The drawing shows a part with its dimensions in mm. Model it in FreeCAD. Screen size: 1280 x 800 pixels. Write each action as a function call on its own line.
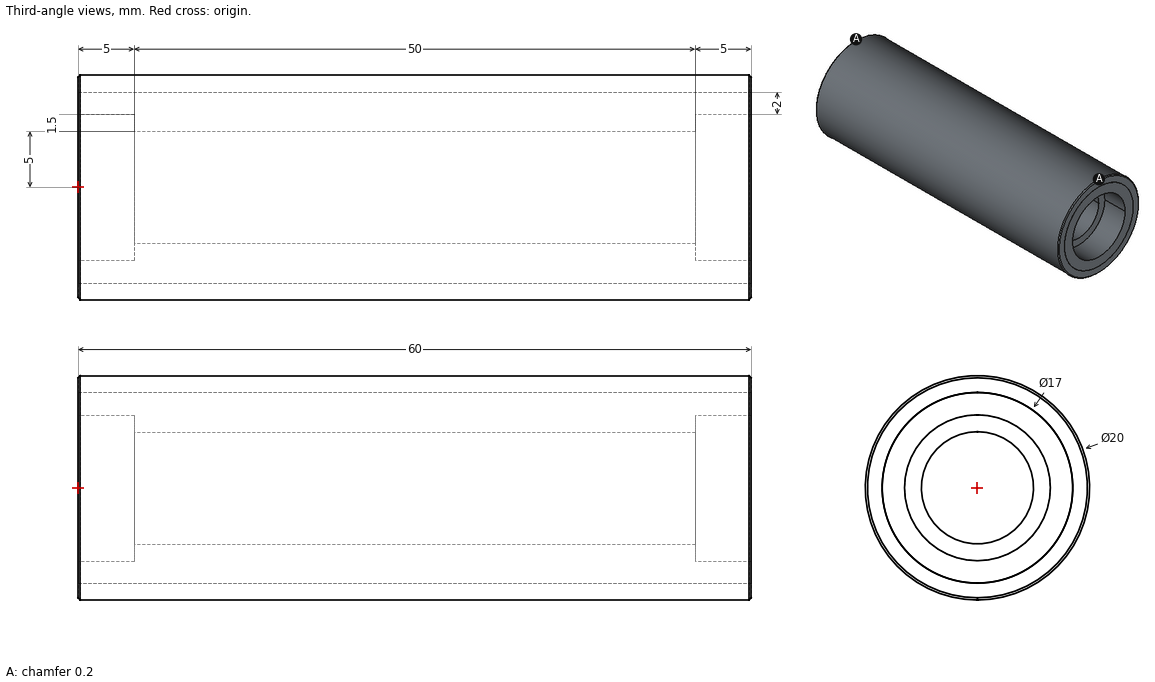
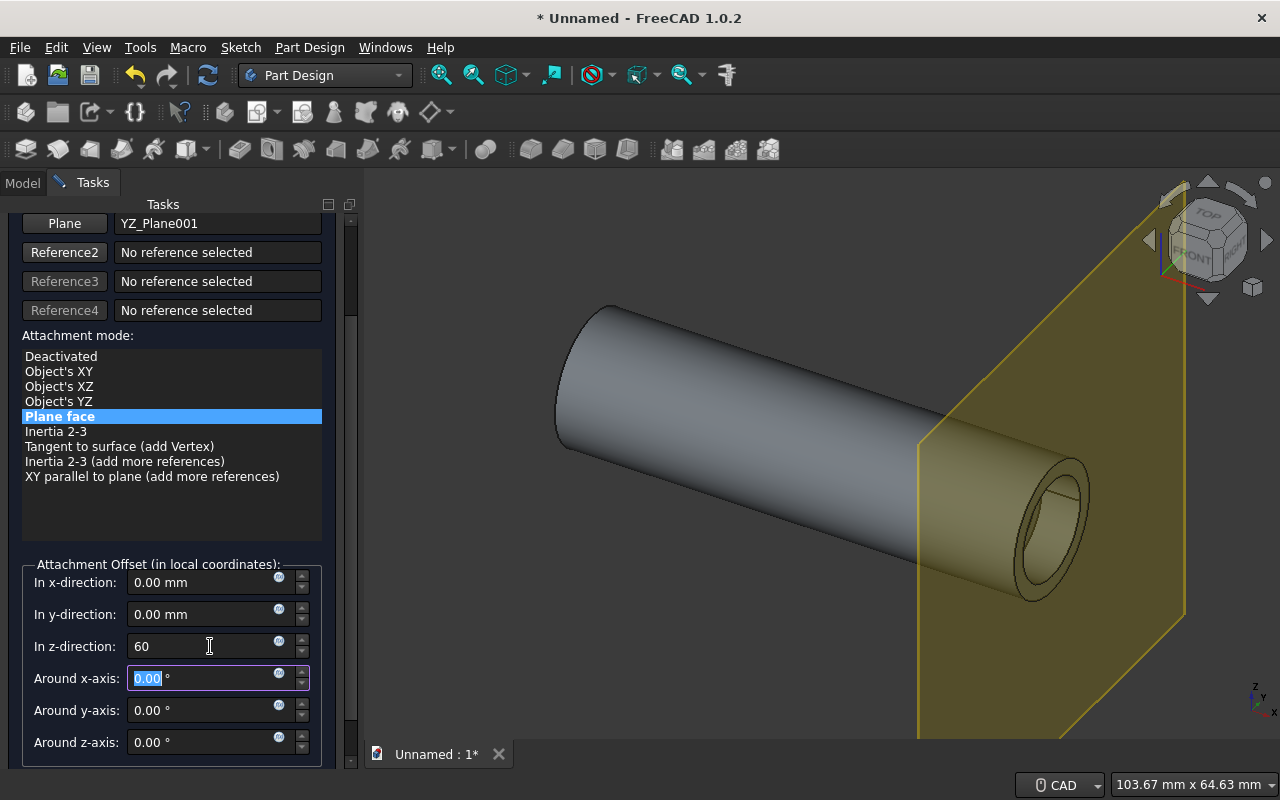
scroll(351, 491, up, 3)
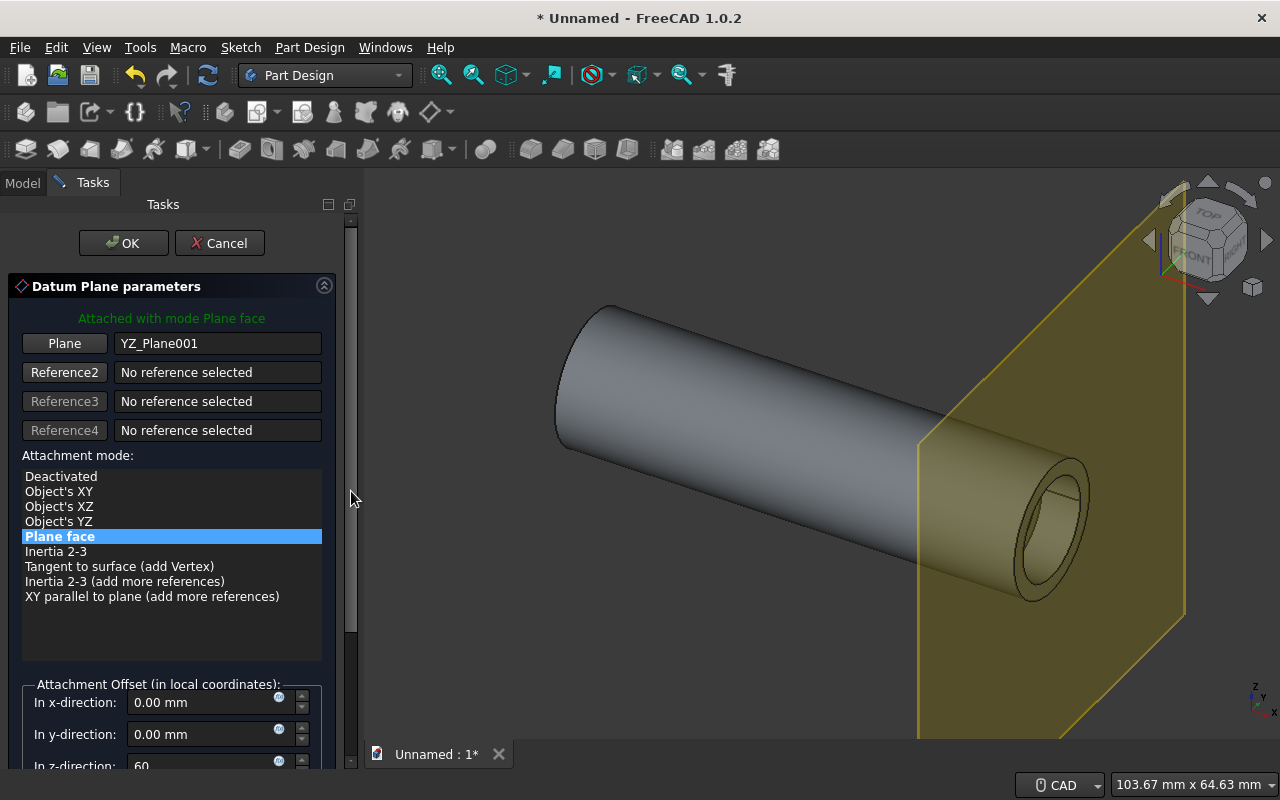
click(124, 243)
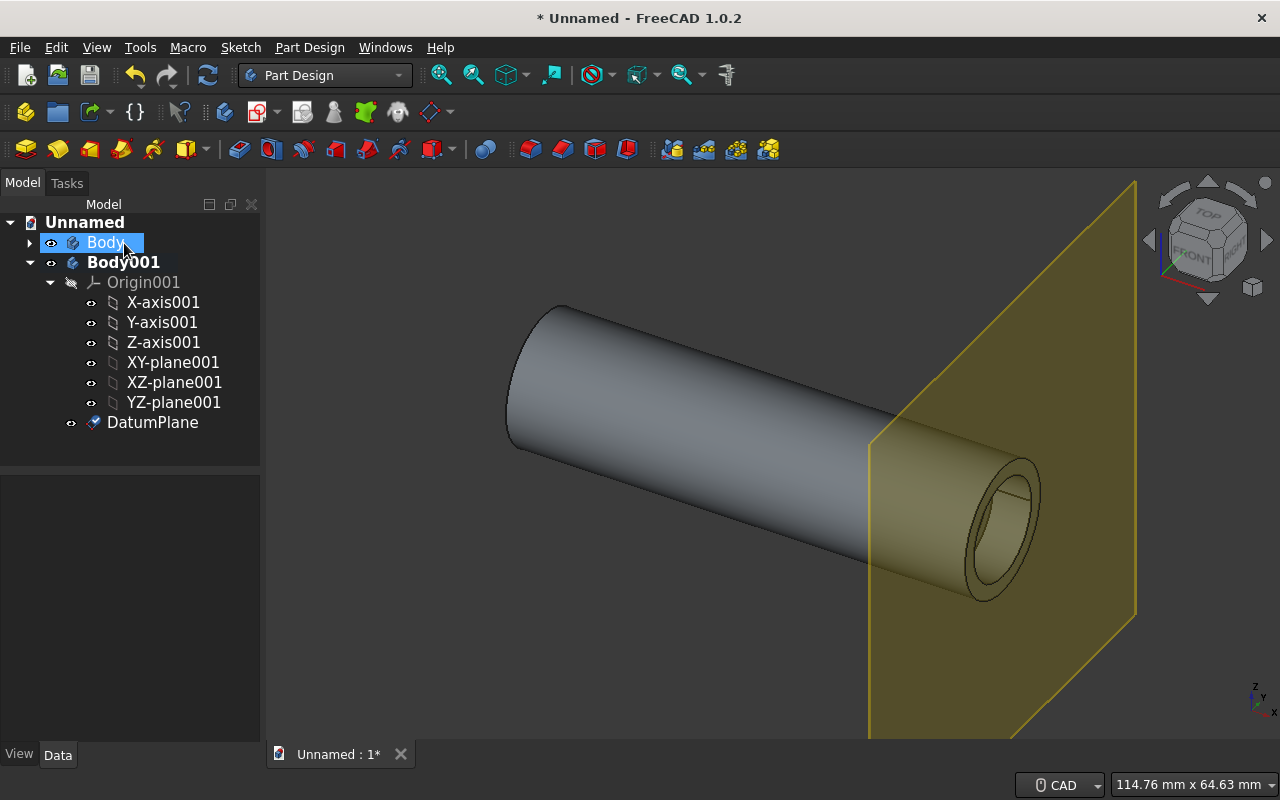
click(116, 423)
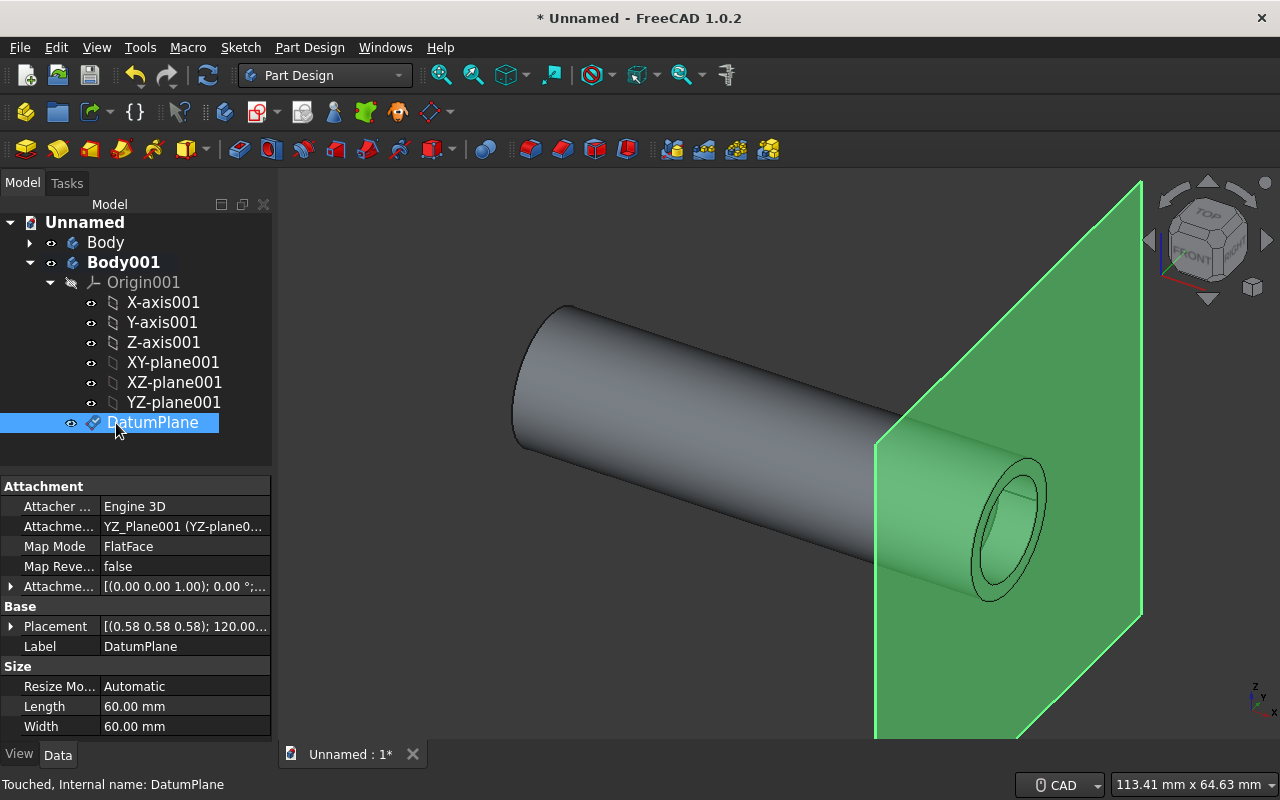
click(258, 112)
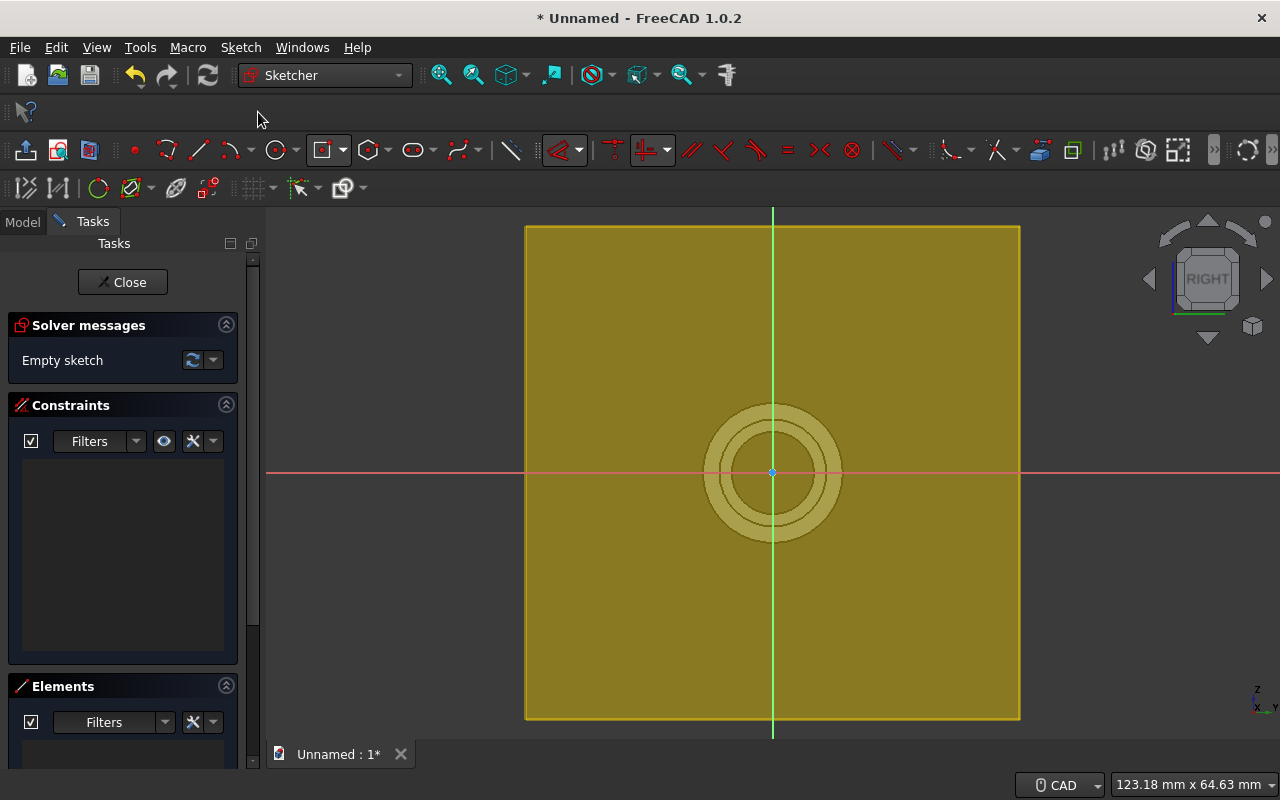
scroll(829, 473, up, 4)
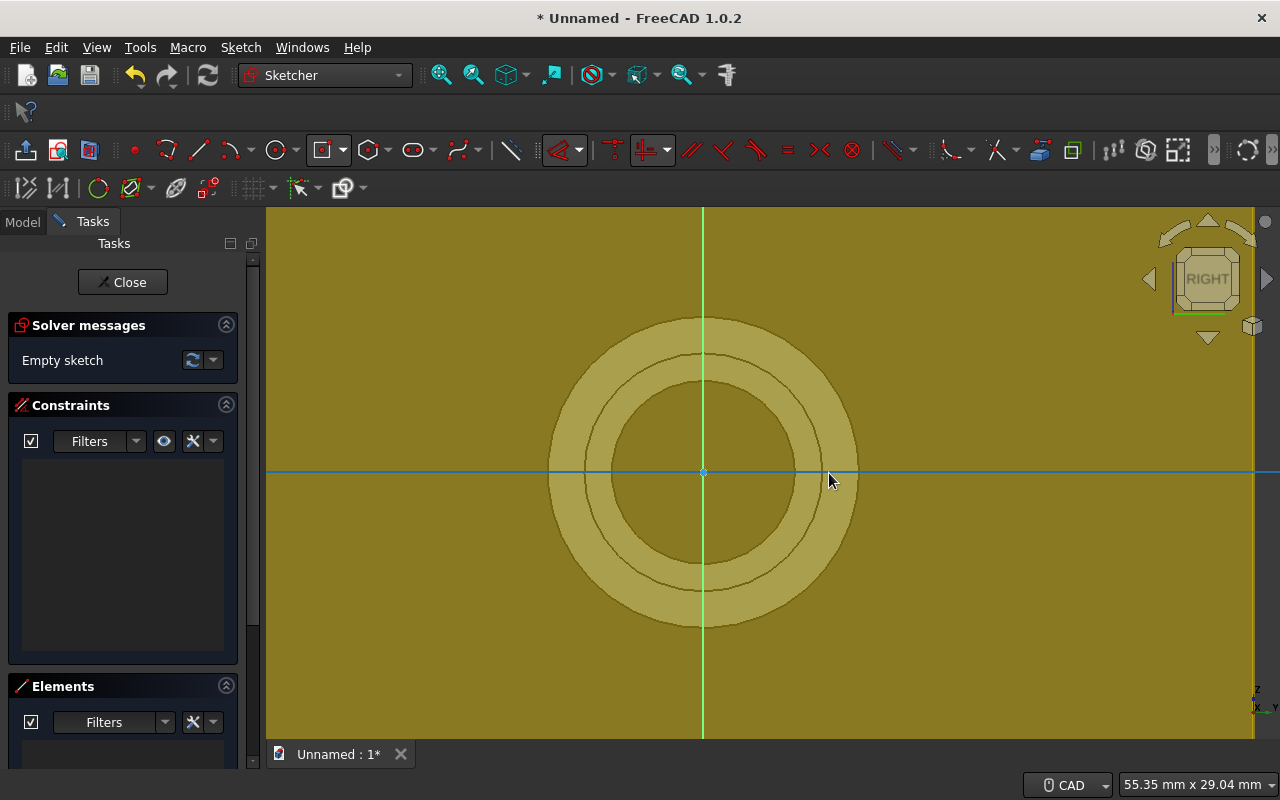
click(276, 150)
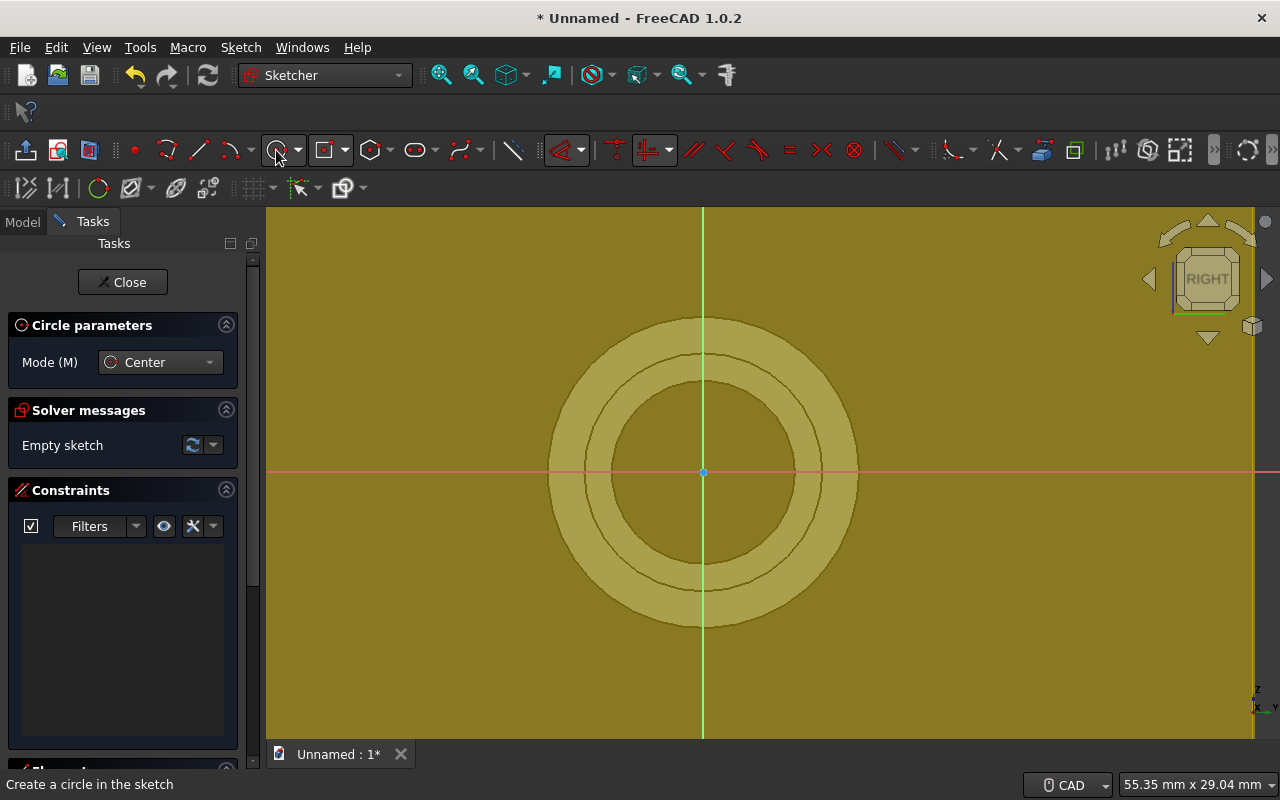
click(703, 472)
move(833, 343)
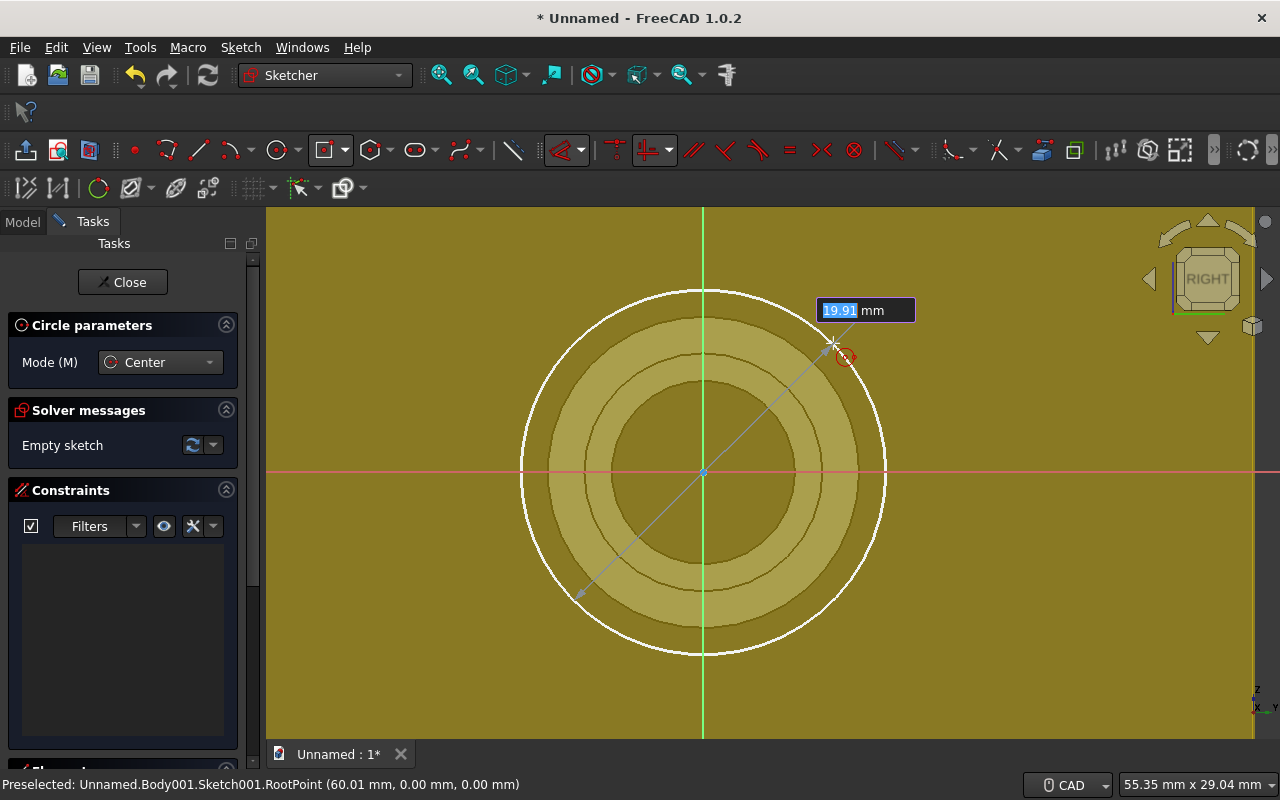
text(20)
key(Return)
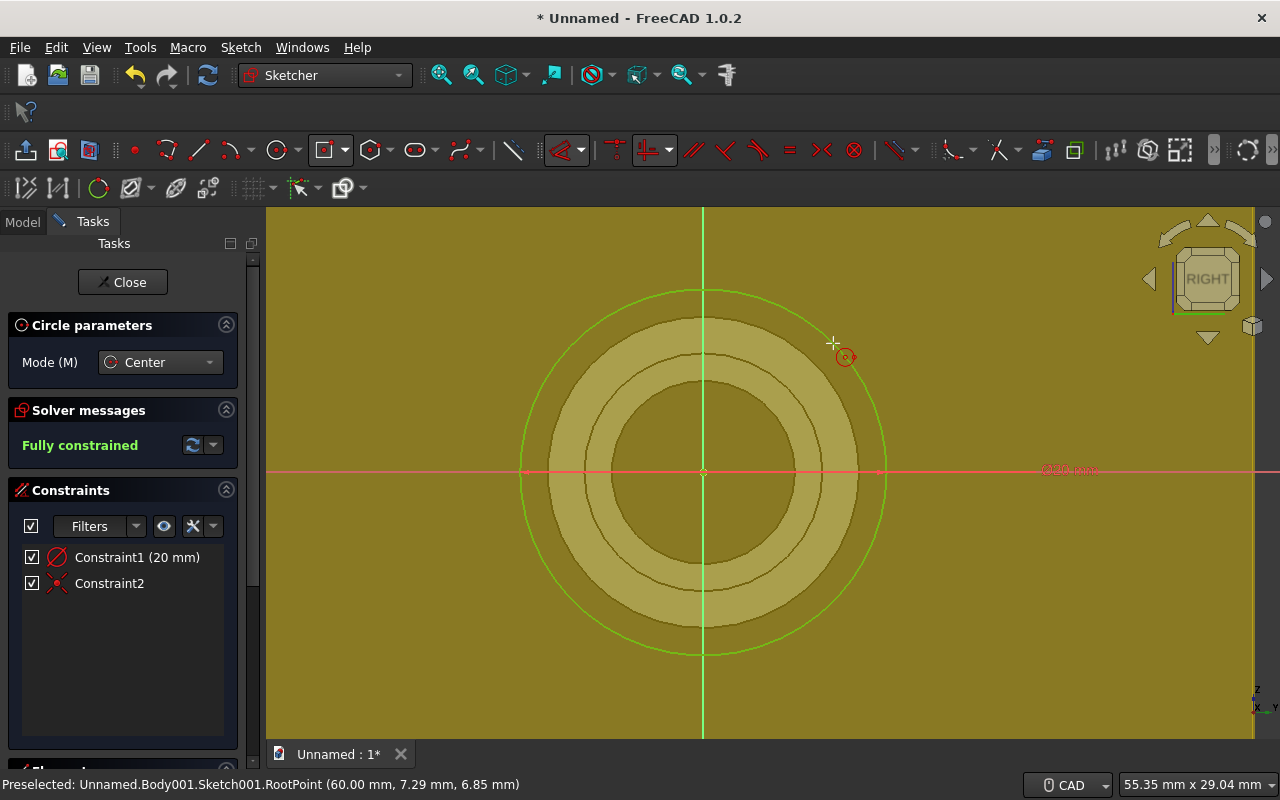
click(703, 472)
move(814, 362)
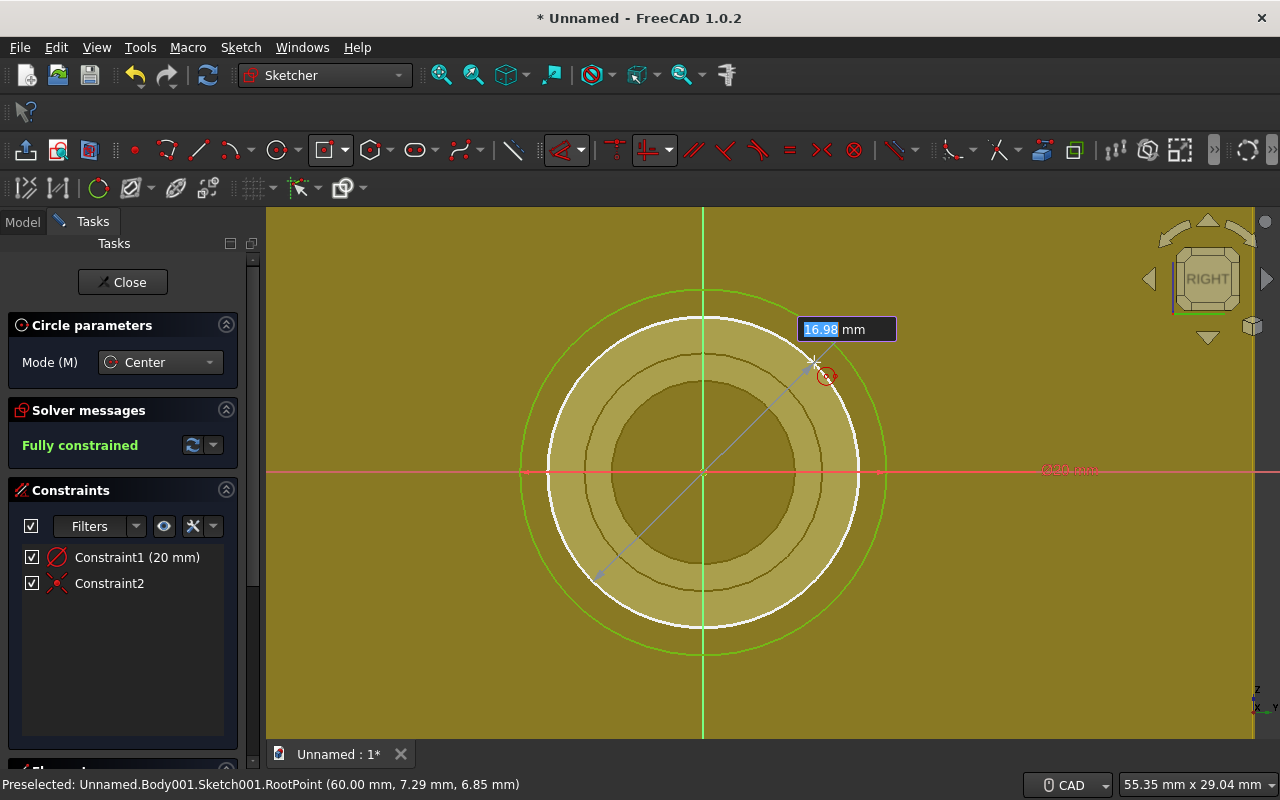
text(17)
key(Return)
key(Escape)